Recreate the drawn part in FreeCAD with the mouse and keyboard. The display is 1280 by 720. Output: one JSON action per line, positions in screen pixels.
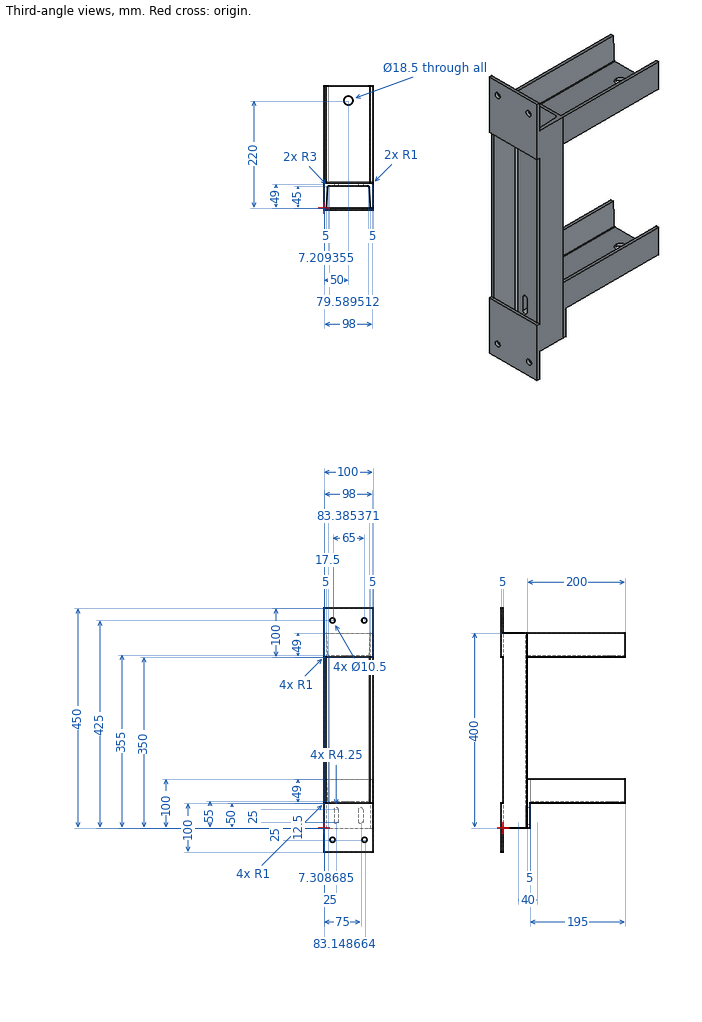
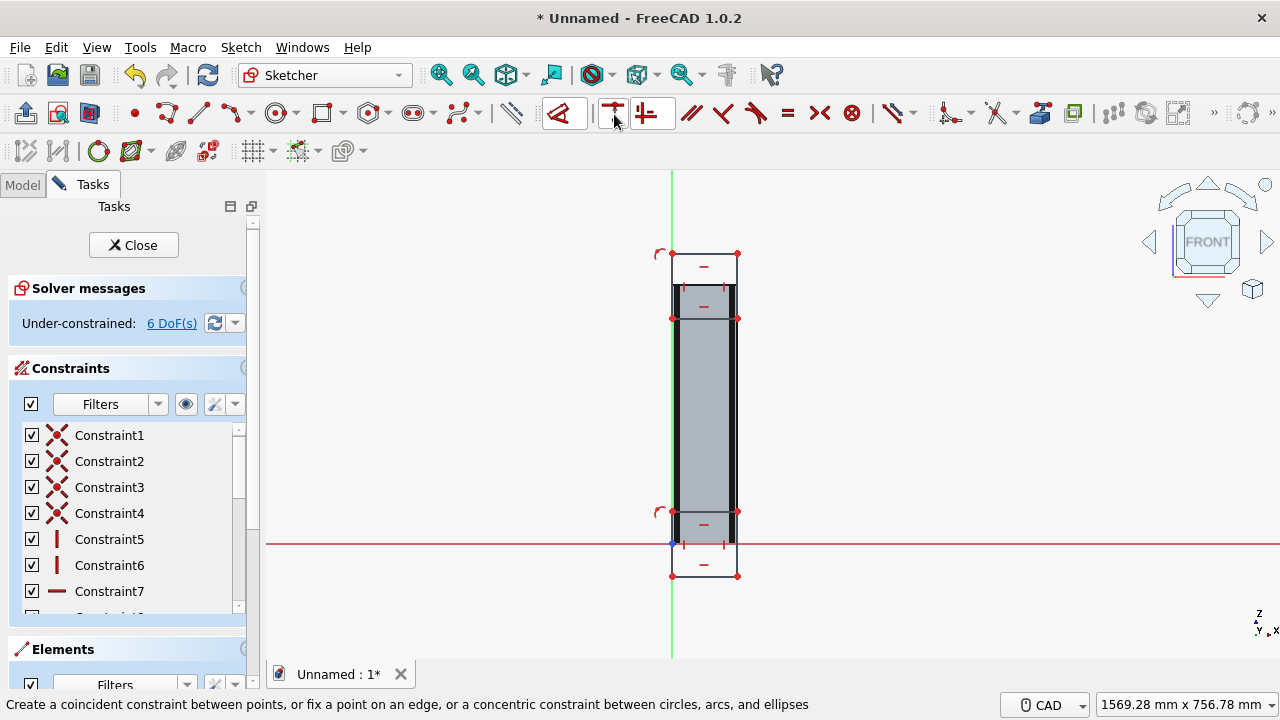
{"action": "left_click", "coordinate": [672, 274]}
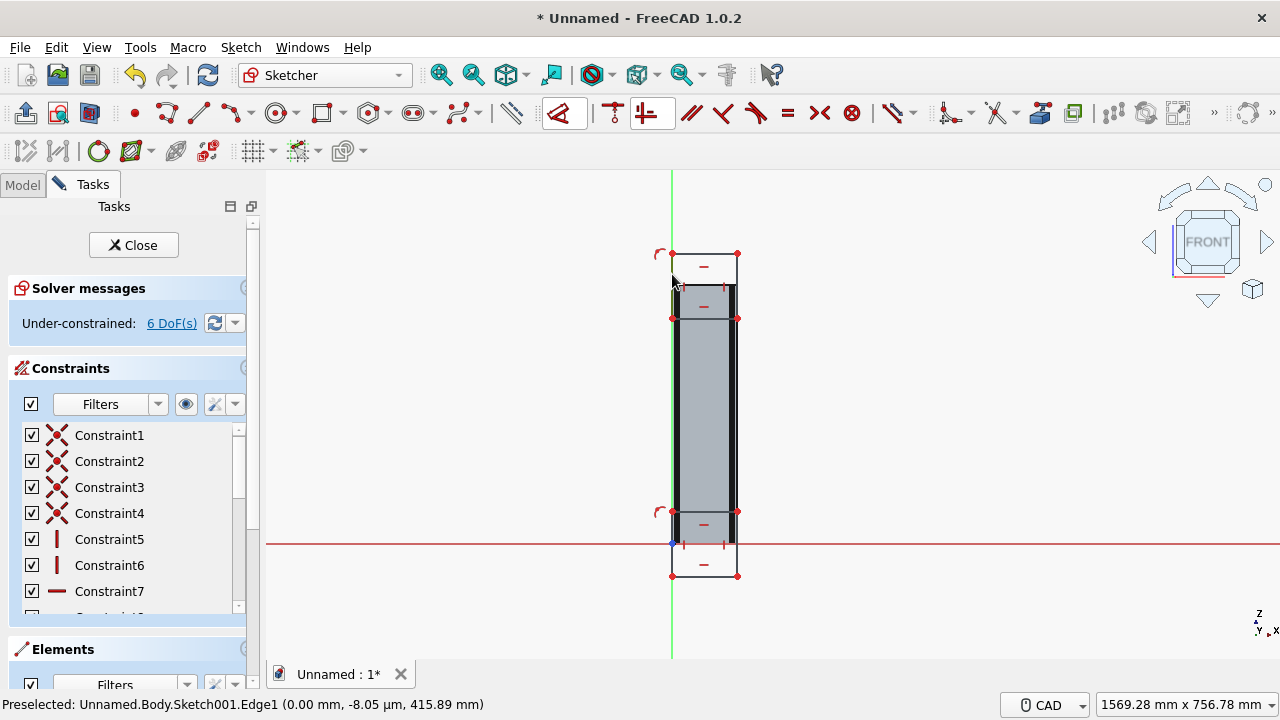
{"action": "key", "text": "i"}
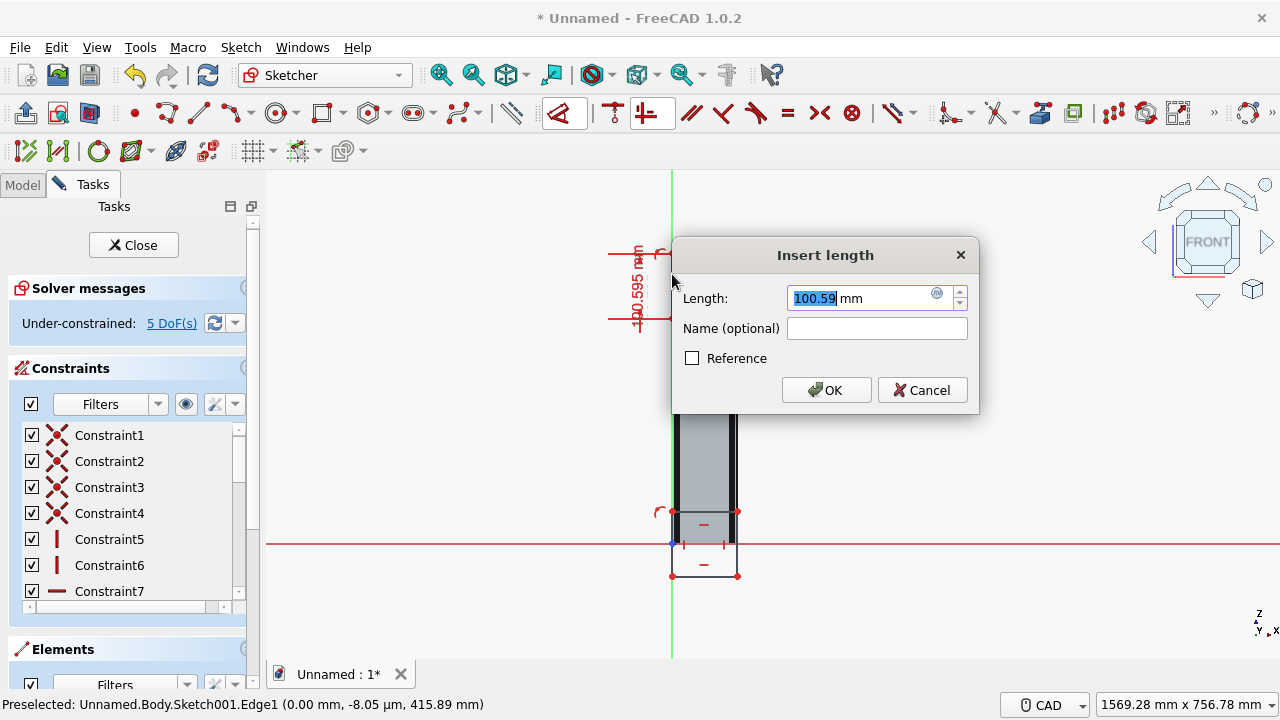
{"action": "type", "text": "100"}
{"action": "key", "text": "Return"}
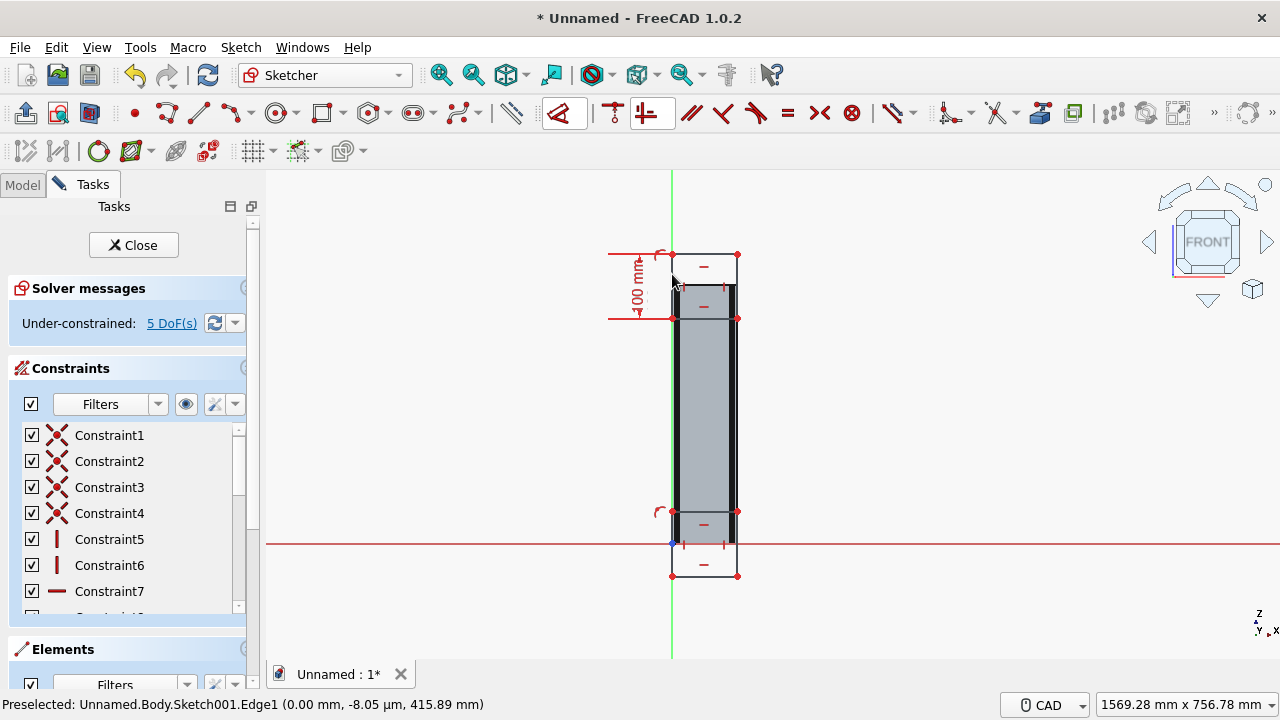
{"action": "left_click", "coordinate": [692, 319]}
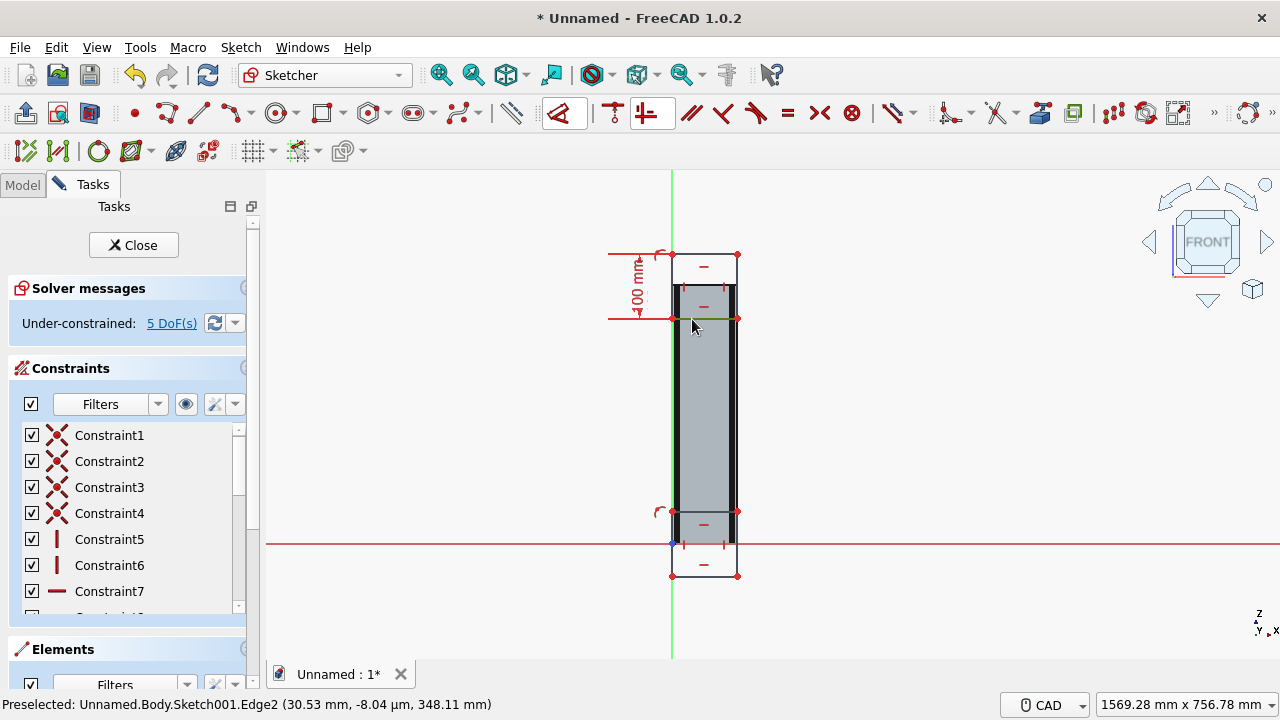
{"action": "key", "text": "l"}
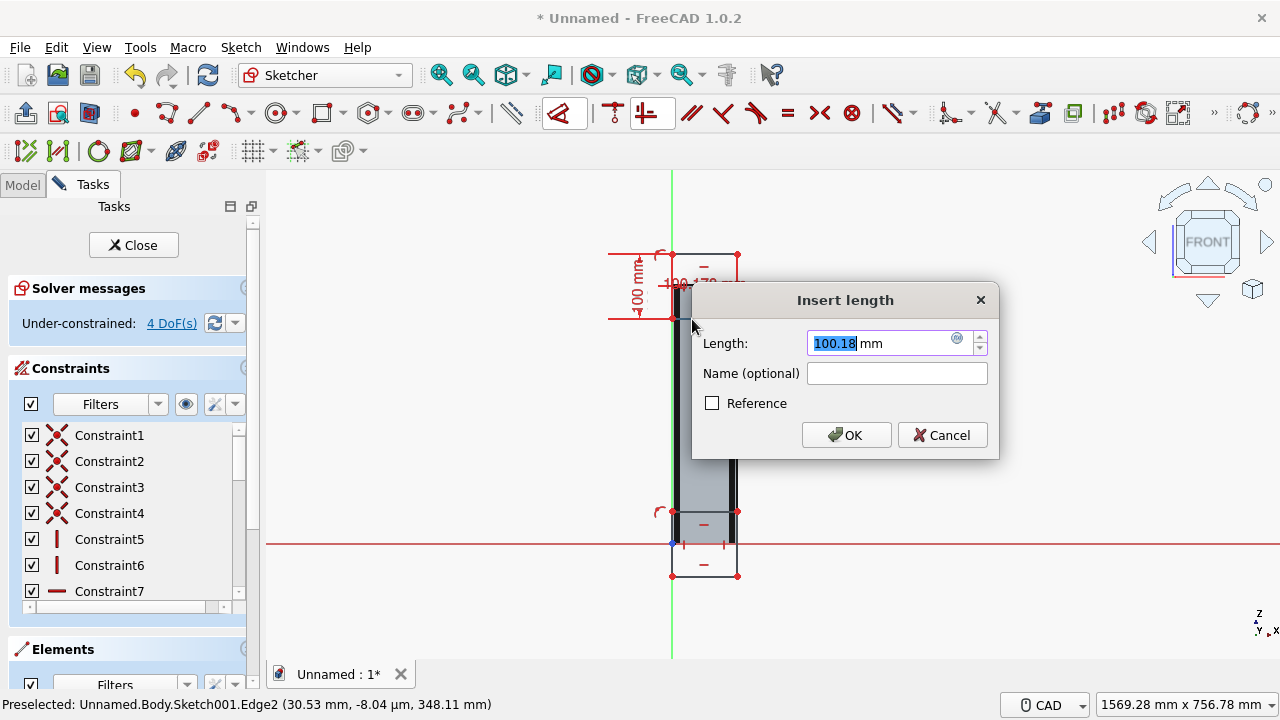
{"action": "type", "text": "100"}
{"action": "key", "text": "Return"}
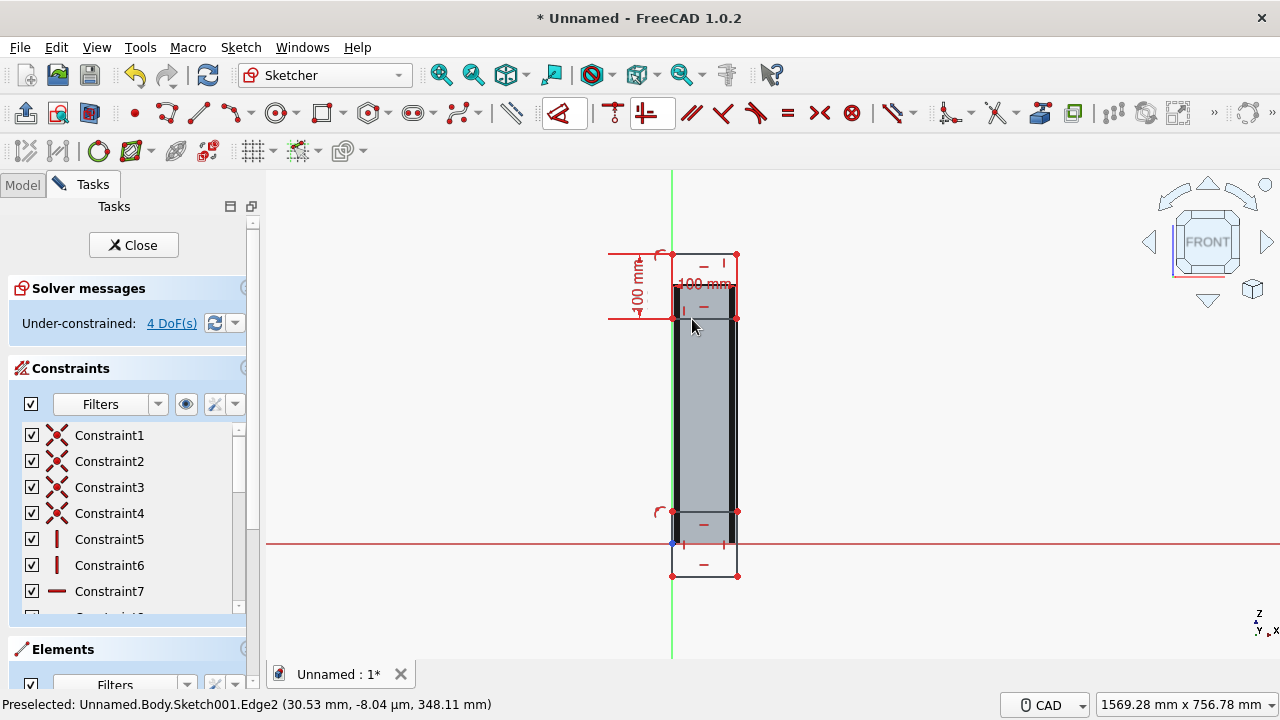
{"action": "left_click", "coordinate": [672, 532]}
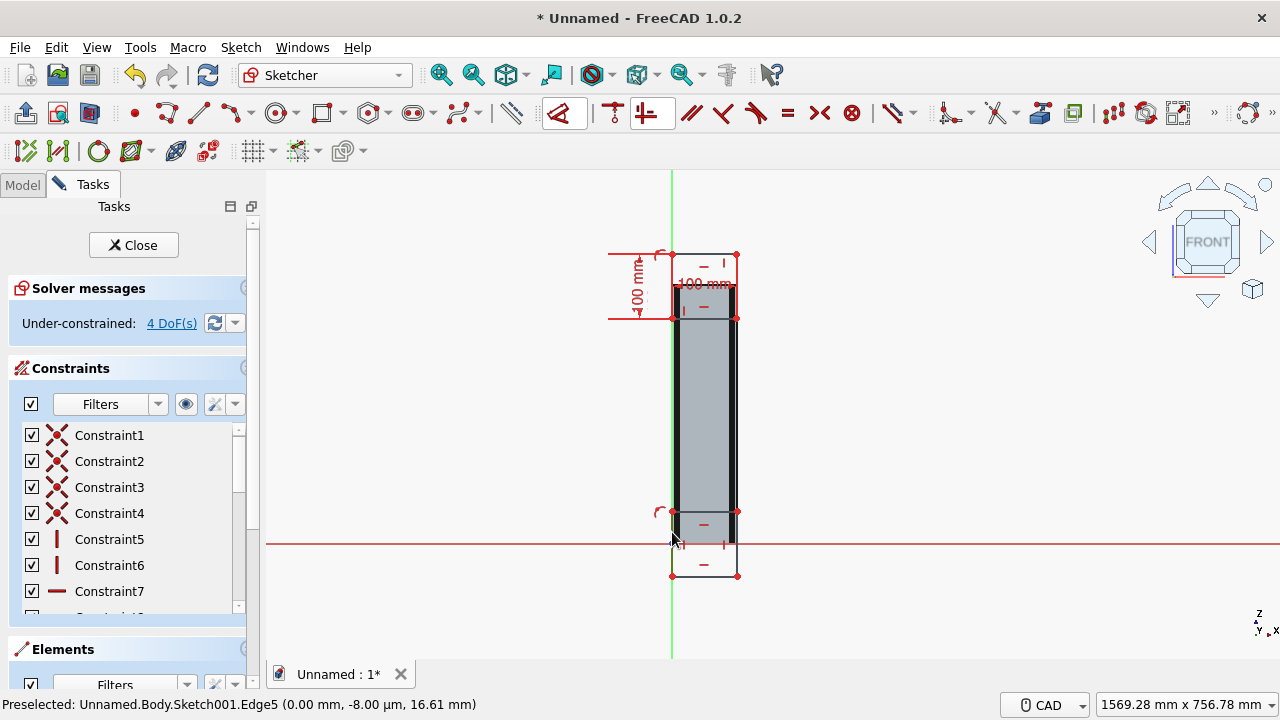
{"action": "left_click", "coordinate": [582, 114]}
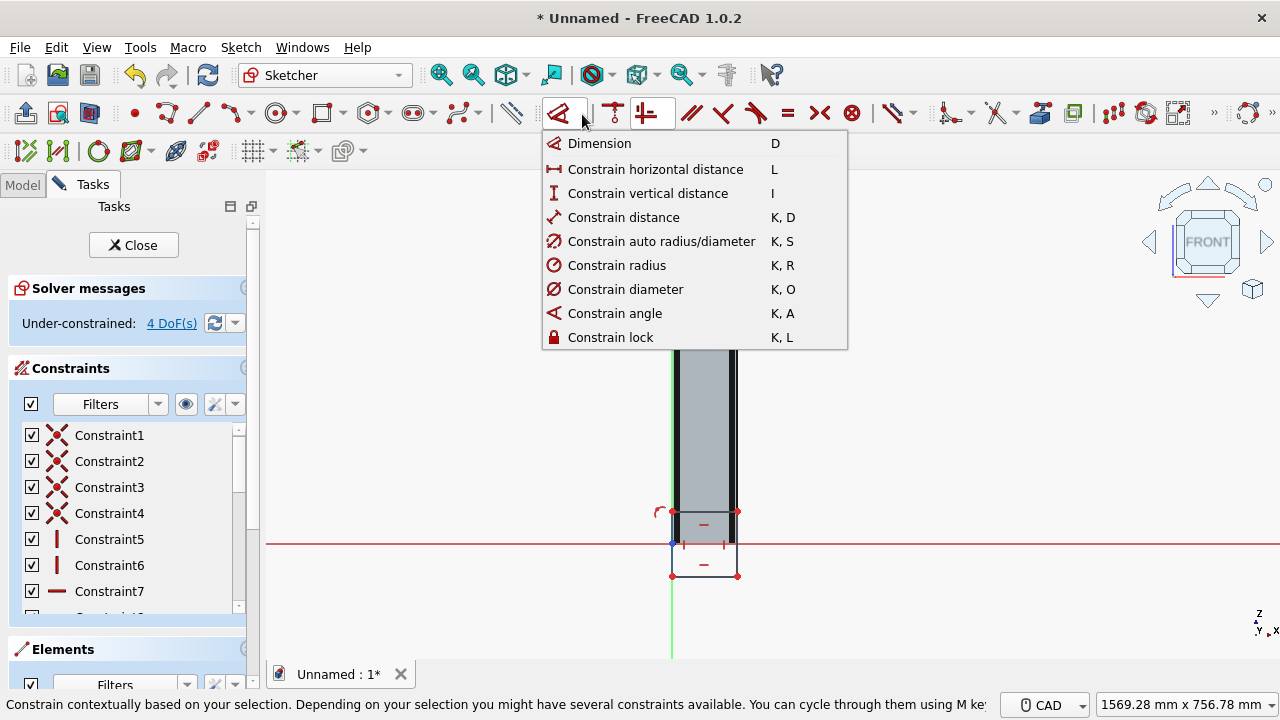
{"action": "left_click", "coordinate": [695, 193]}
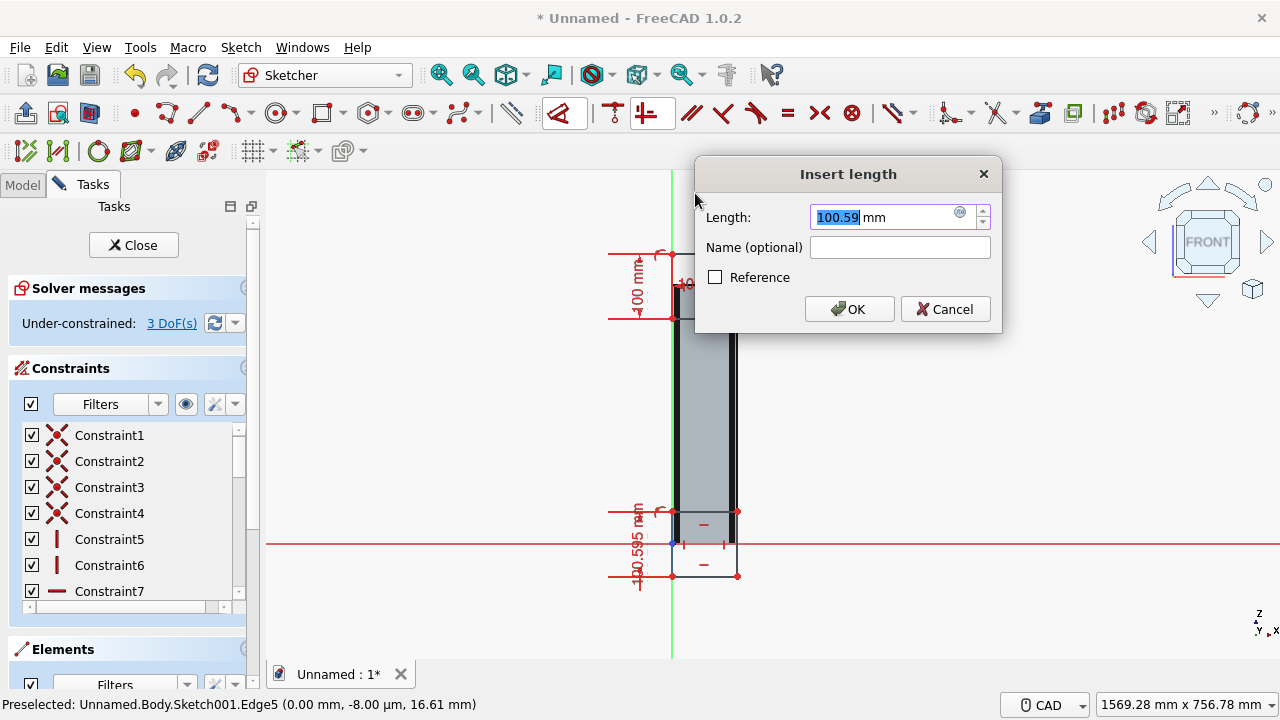
{"action": "type", "text": "100"}
{"action": "key", "text": "Return"}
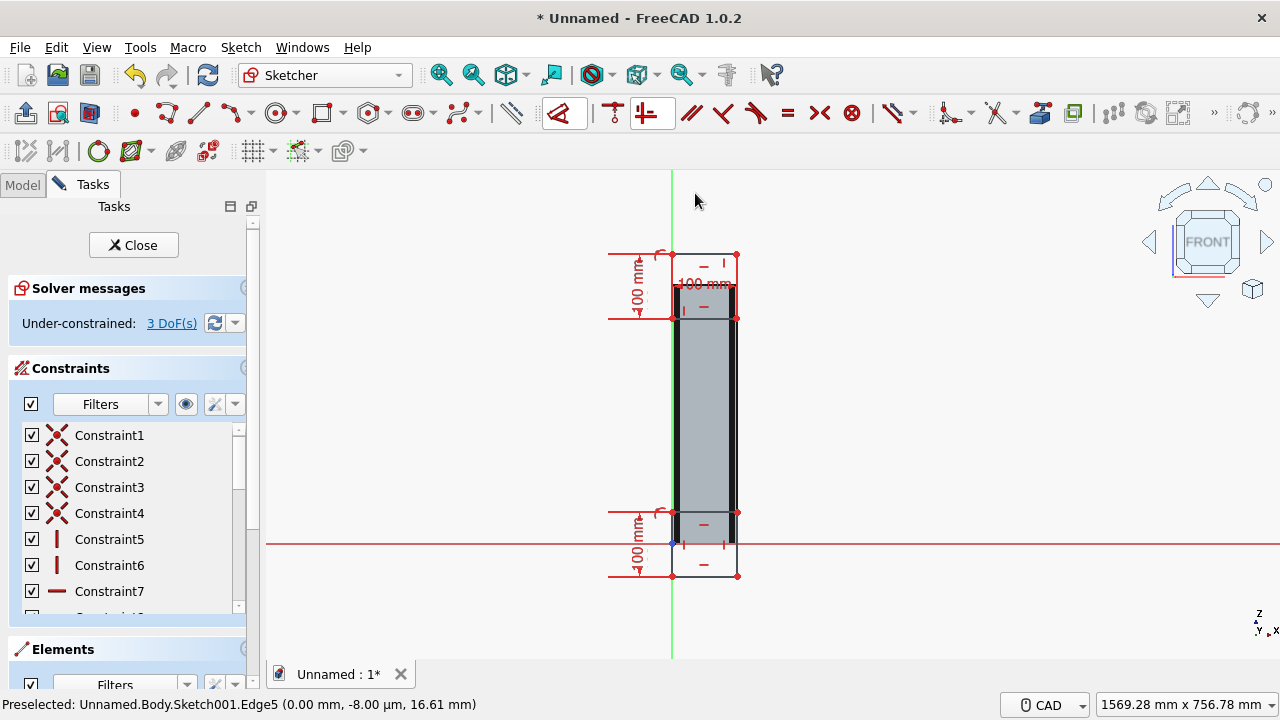
{"action": "left_click", "coordinate": [692, 577]}